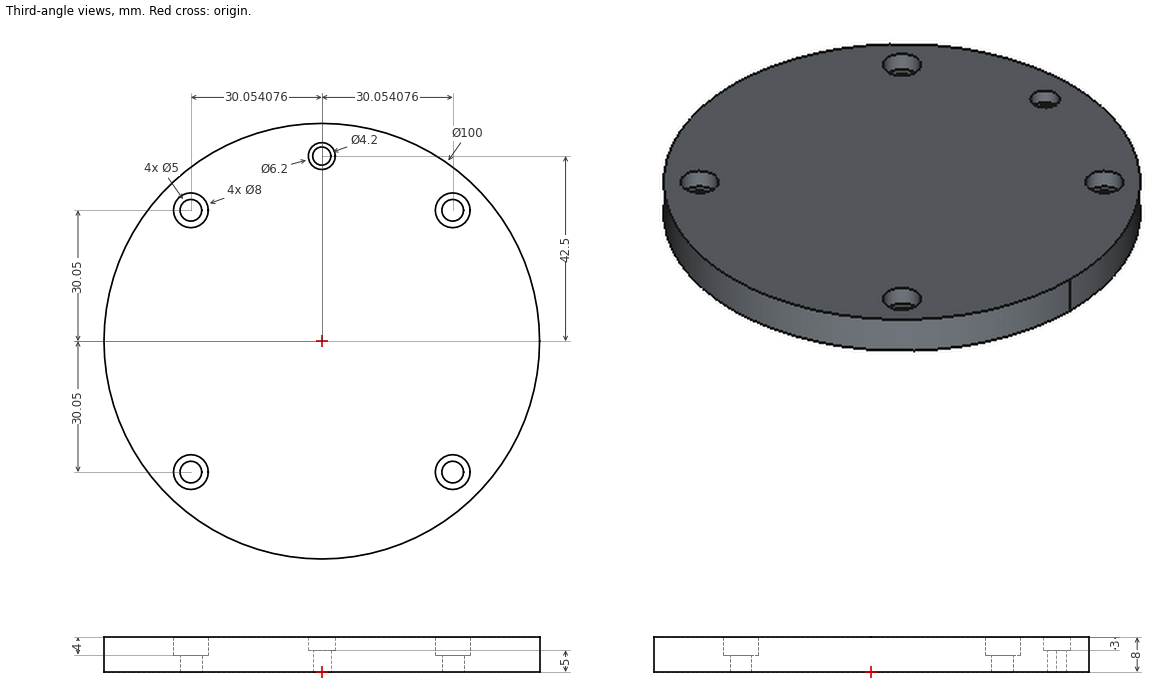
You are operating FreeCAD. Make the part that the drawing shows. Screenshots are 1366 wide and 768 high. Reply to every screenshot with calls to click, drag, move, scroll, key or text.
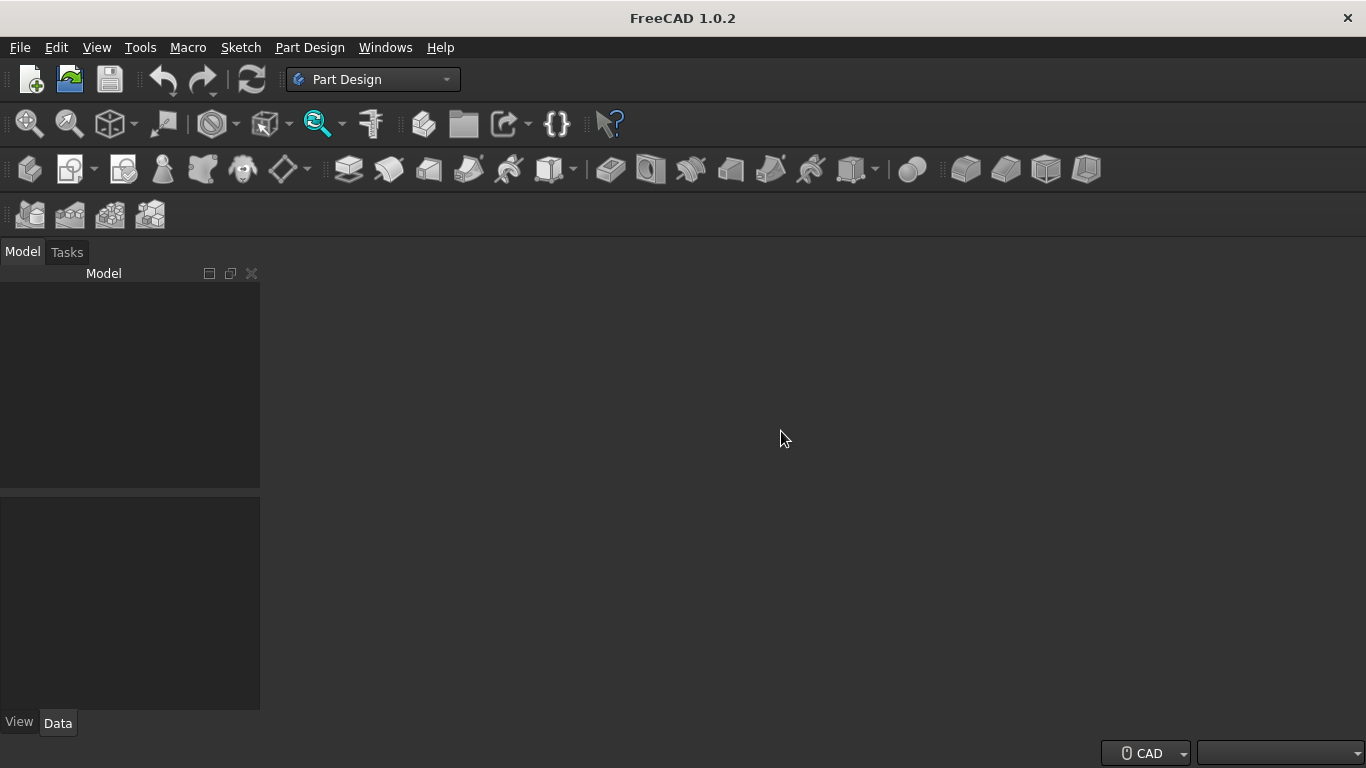
click(30, 80)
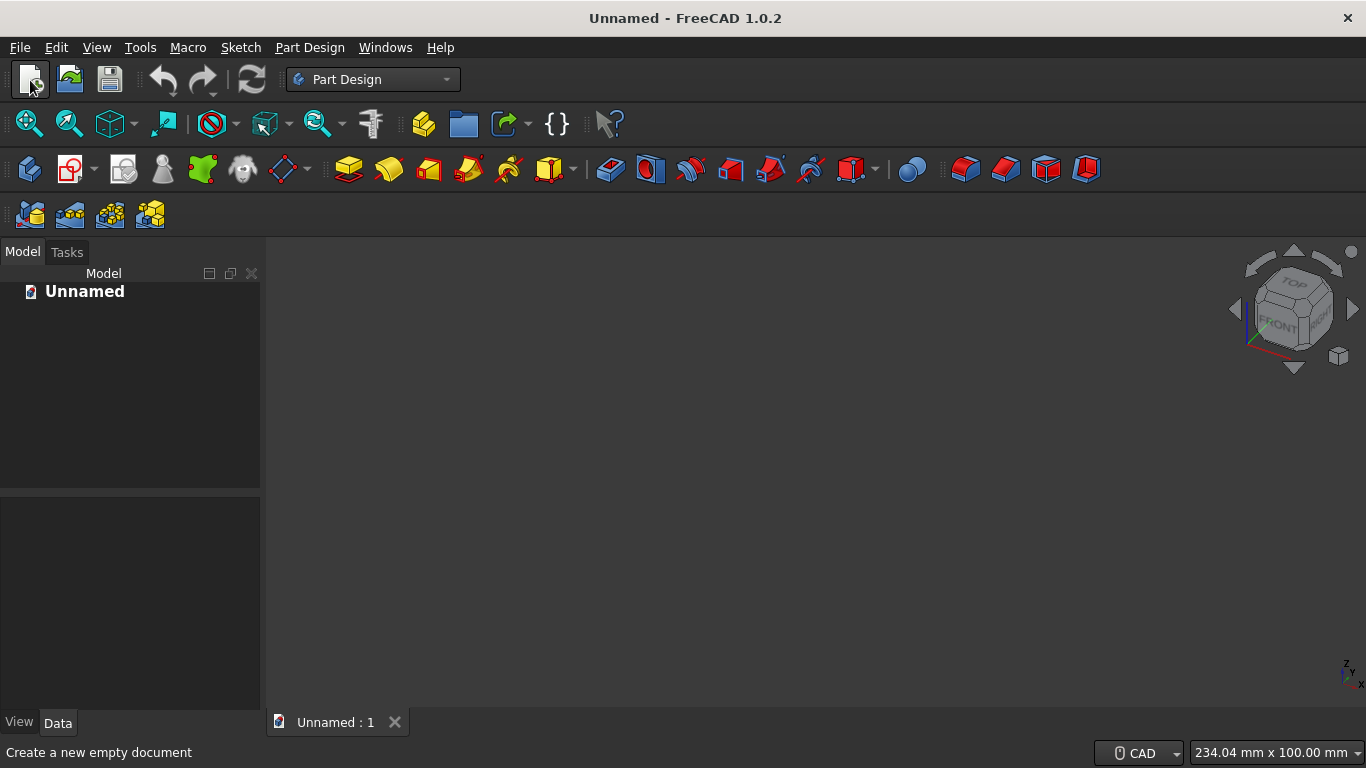
click(70, 170)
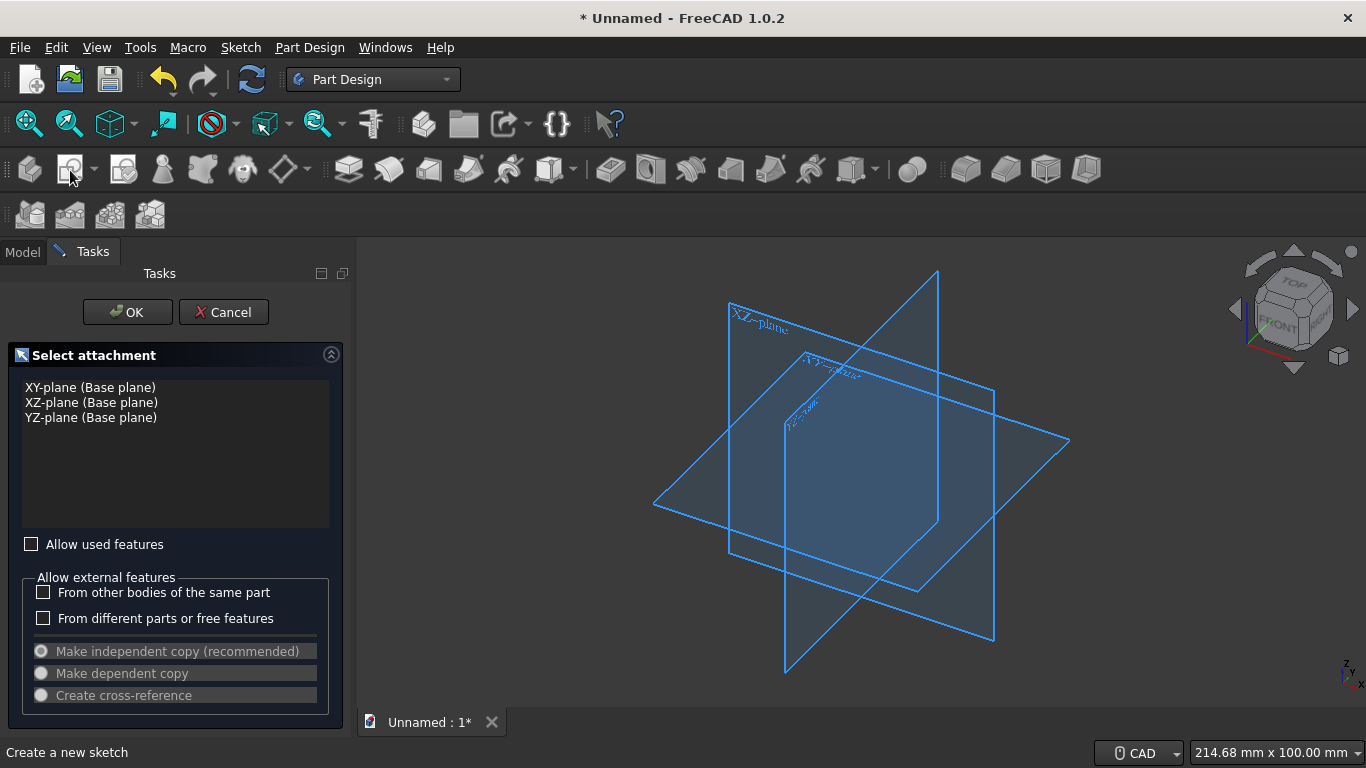
click(82, 388)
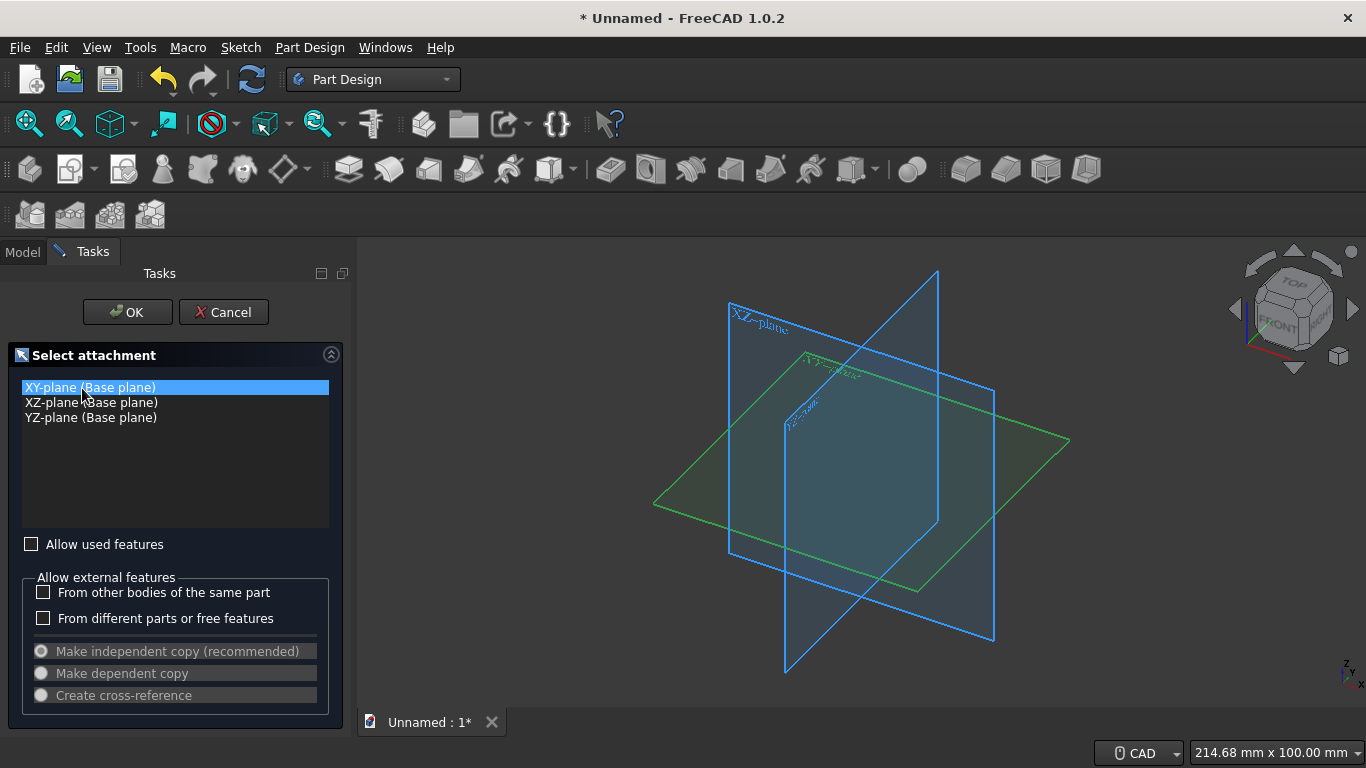
click(128, 312)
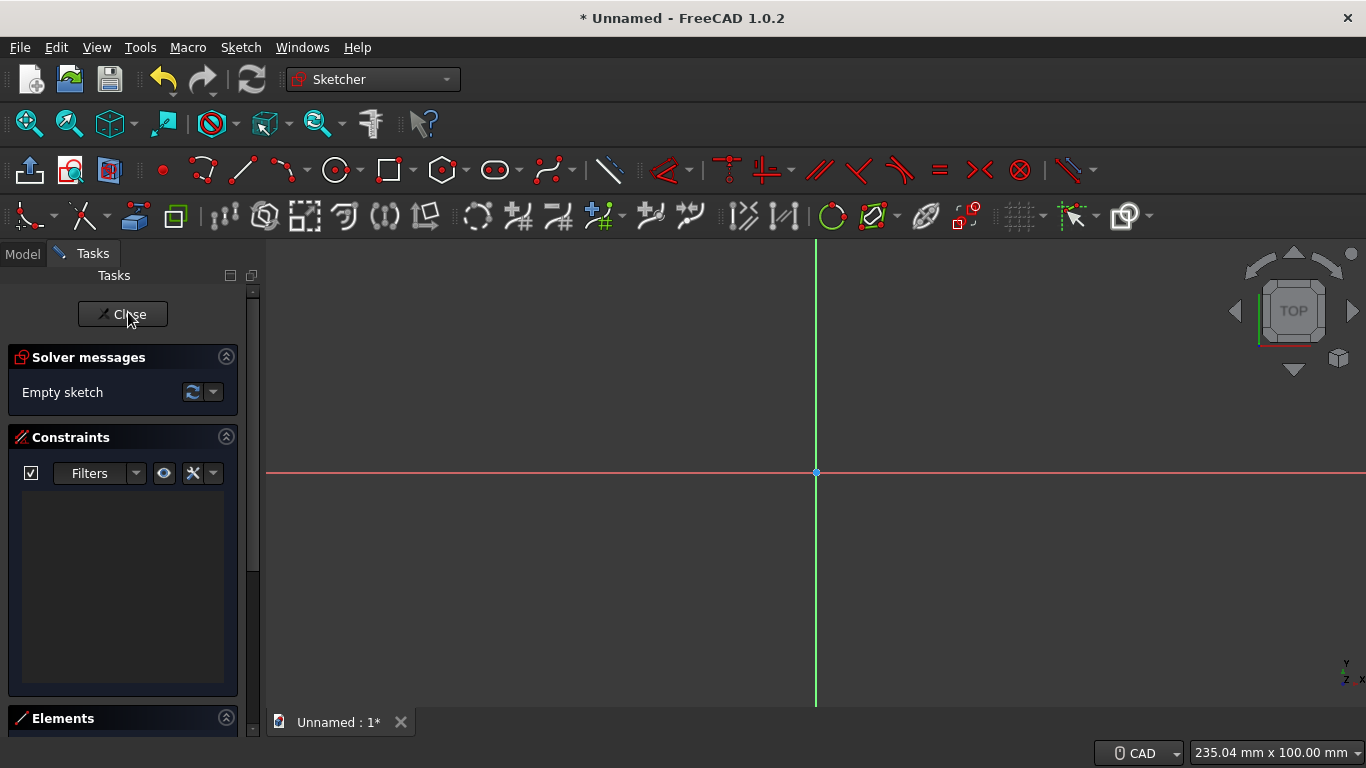
scroll(608, 473, down, 2)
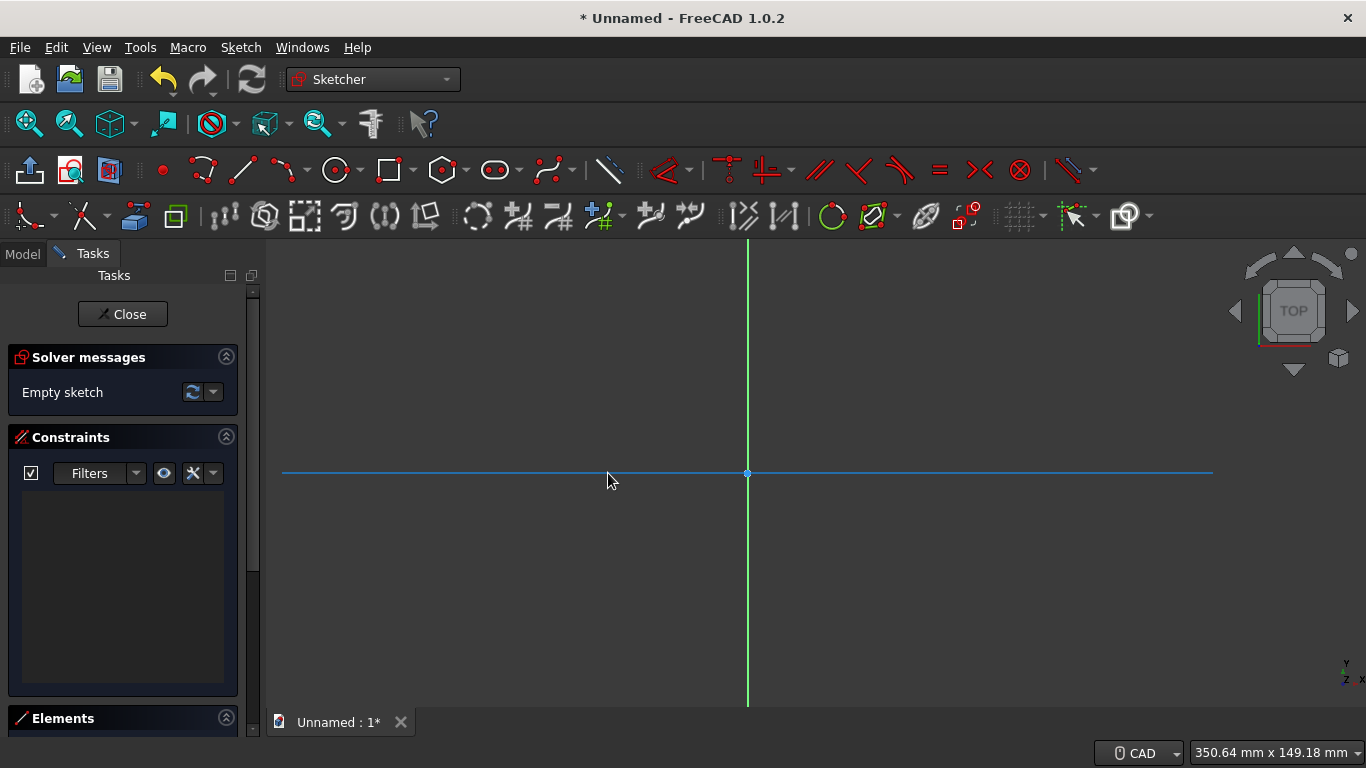
click(336, 170)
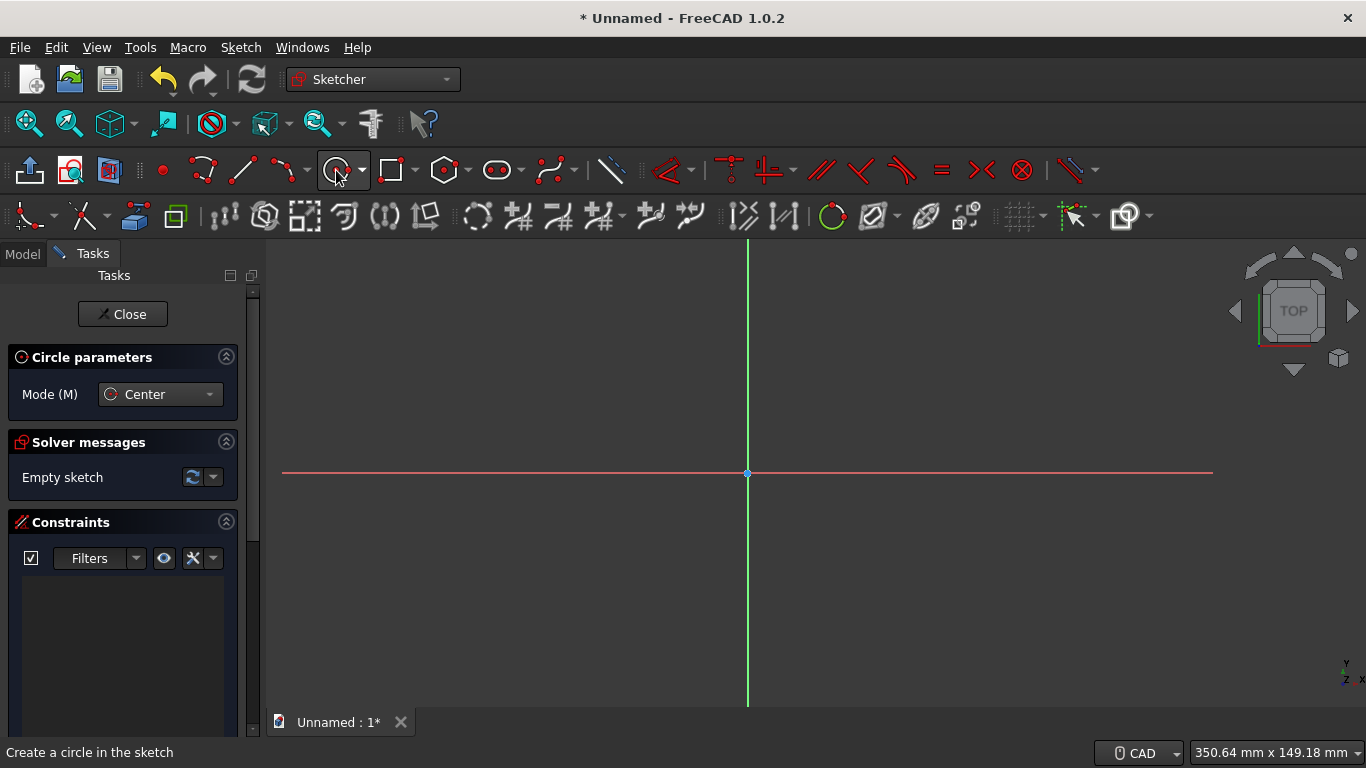
click(748, 473)
move(858, 362)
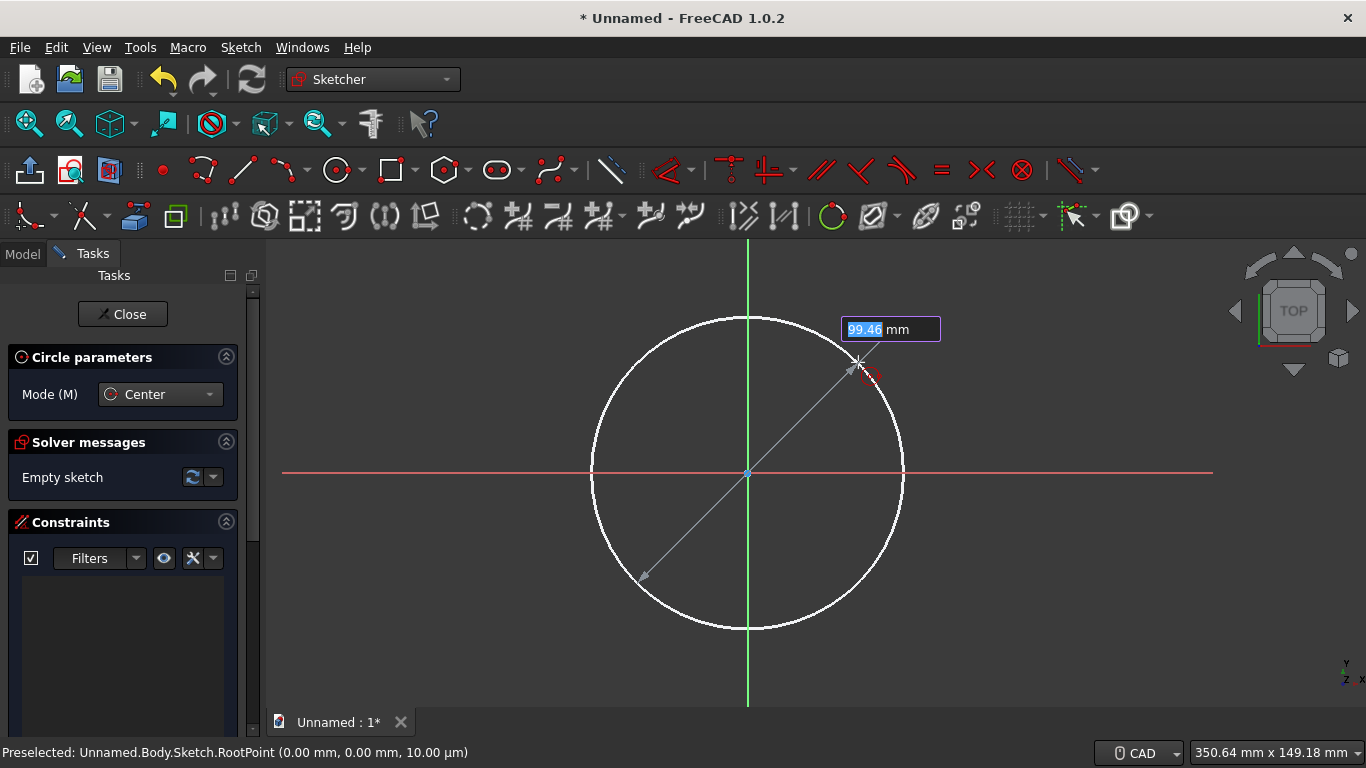
text(100)
key(Return)
key(Escape)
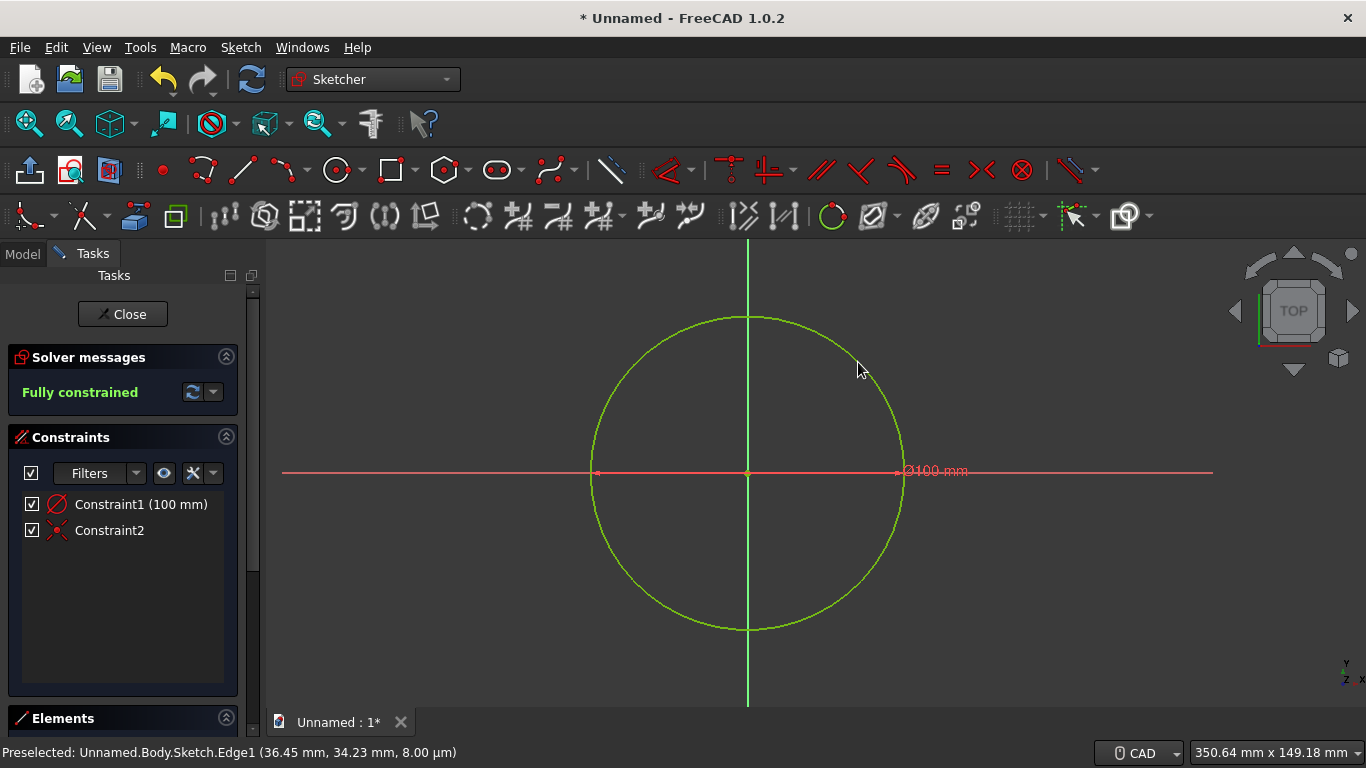
click(123, 314)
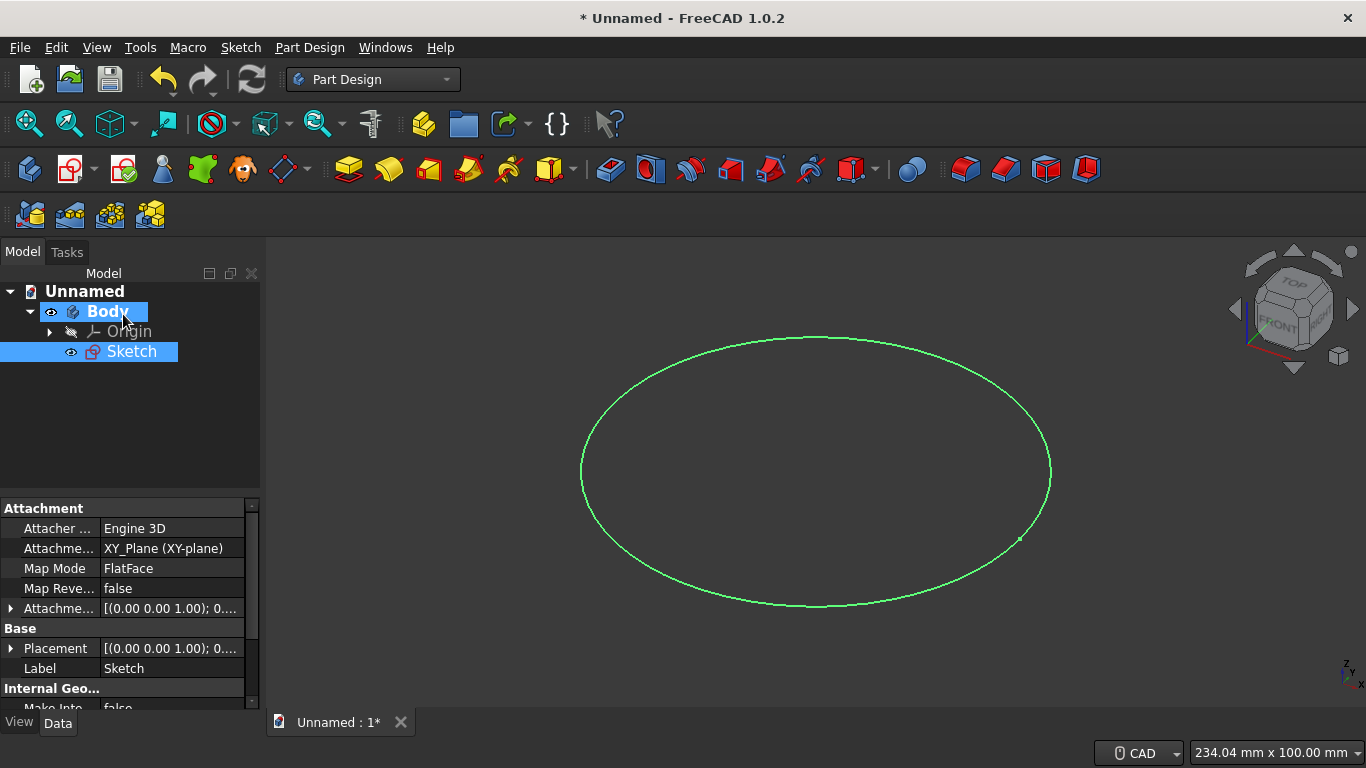
click(350, 170)